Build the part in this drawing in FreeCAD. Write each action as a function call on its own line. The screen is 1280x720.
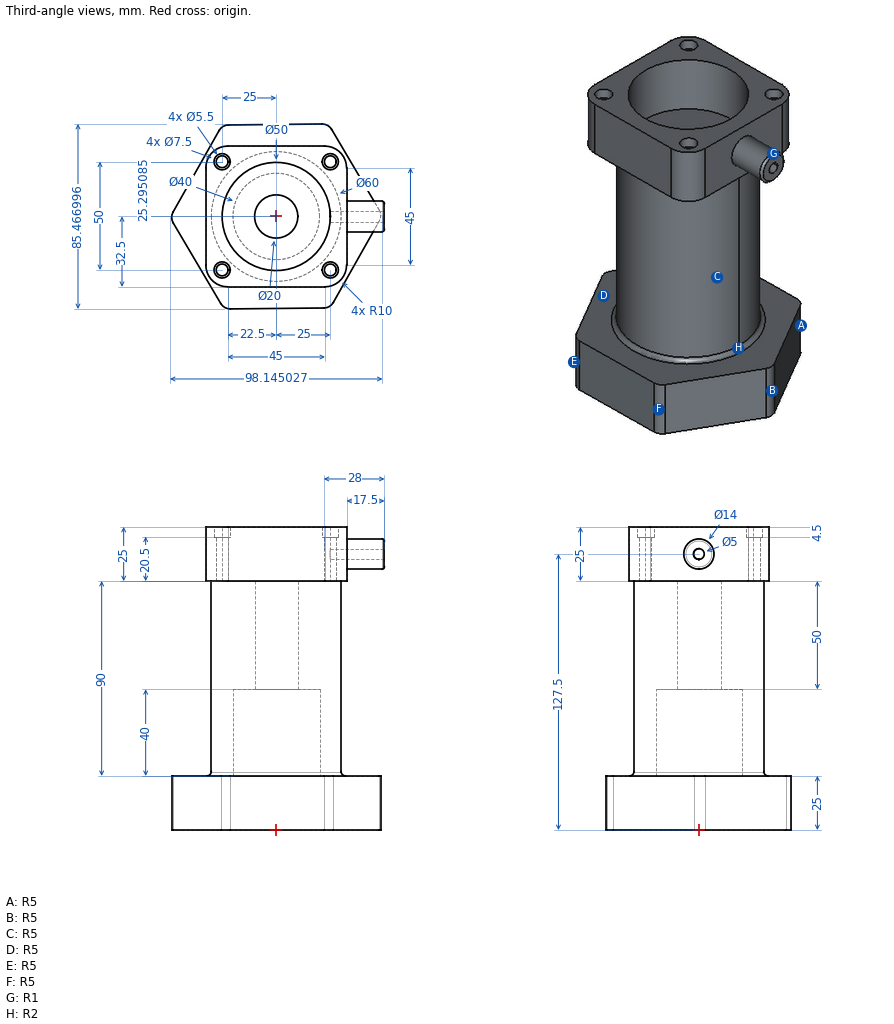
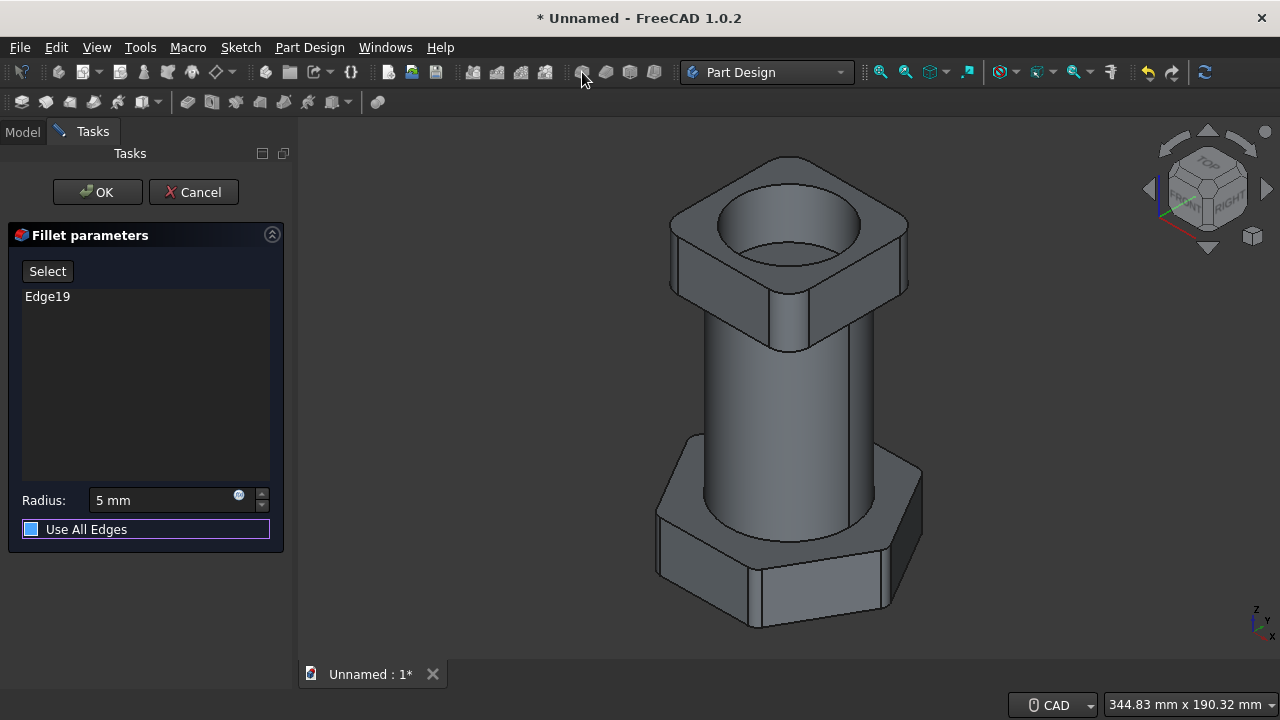
click(98, 192)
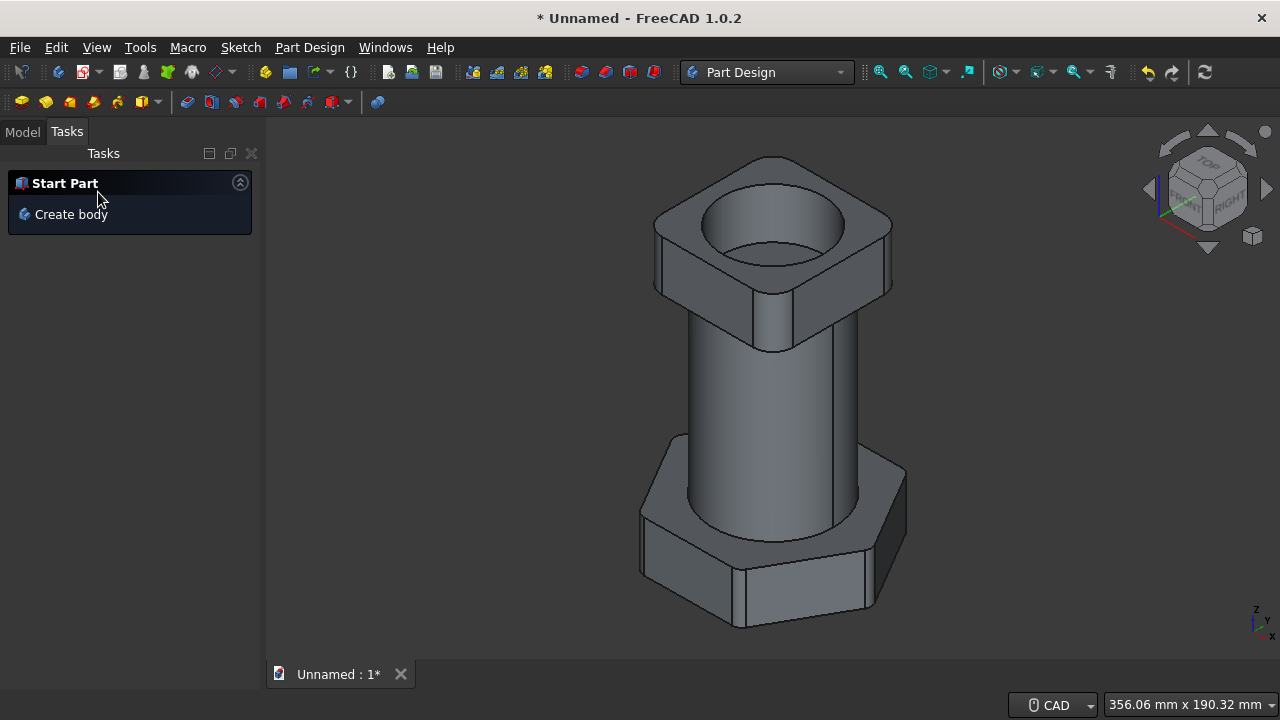
click(867, 235)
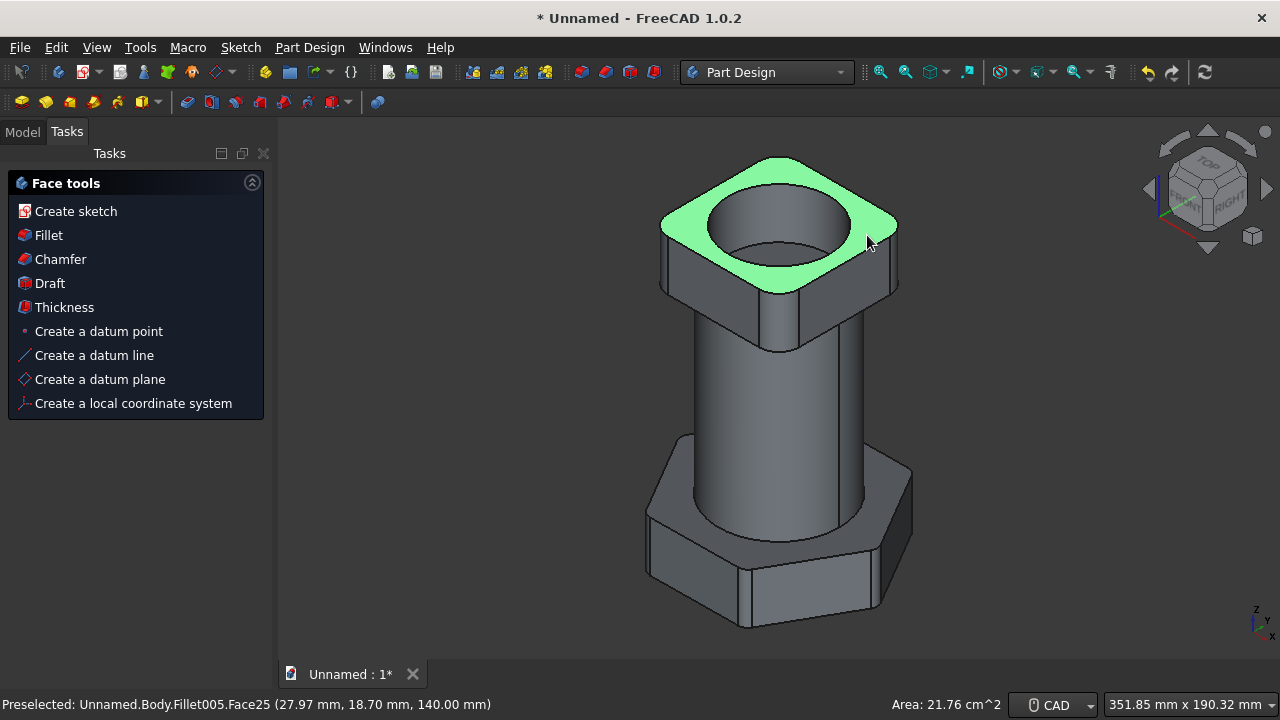
click(84, 72)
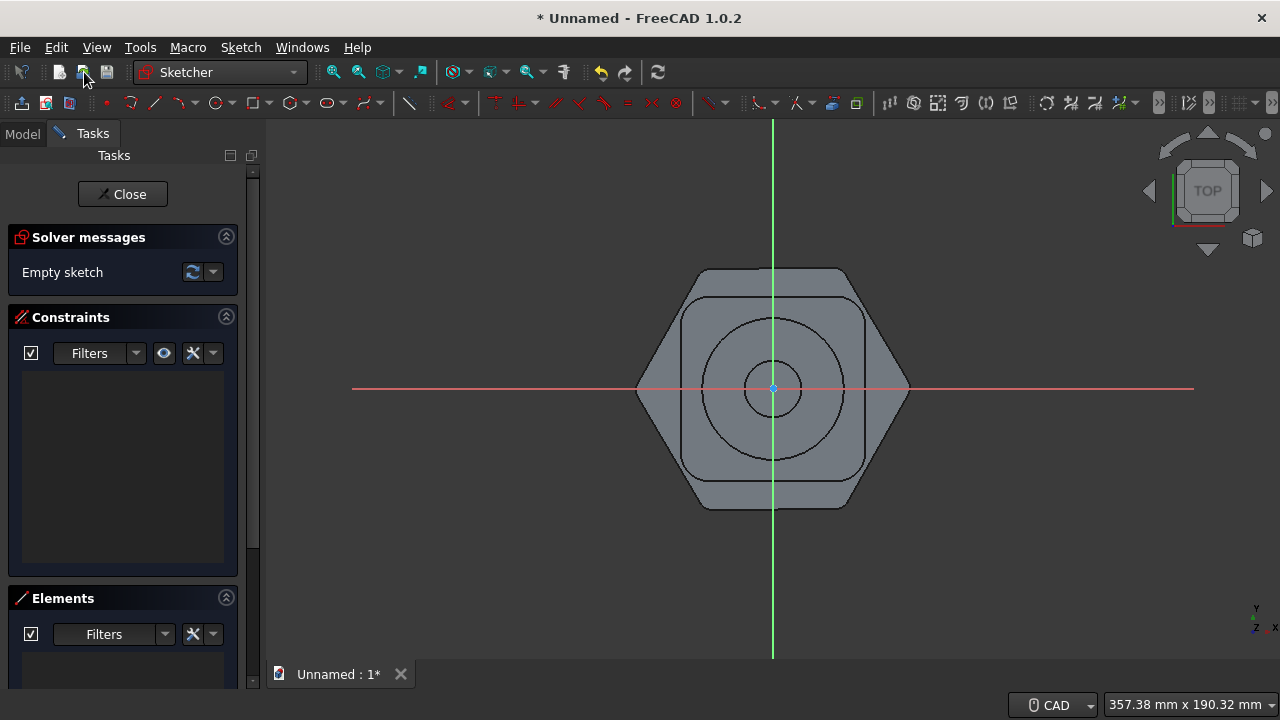
scroll(829, 387, up, 4)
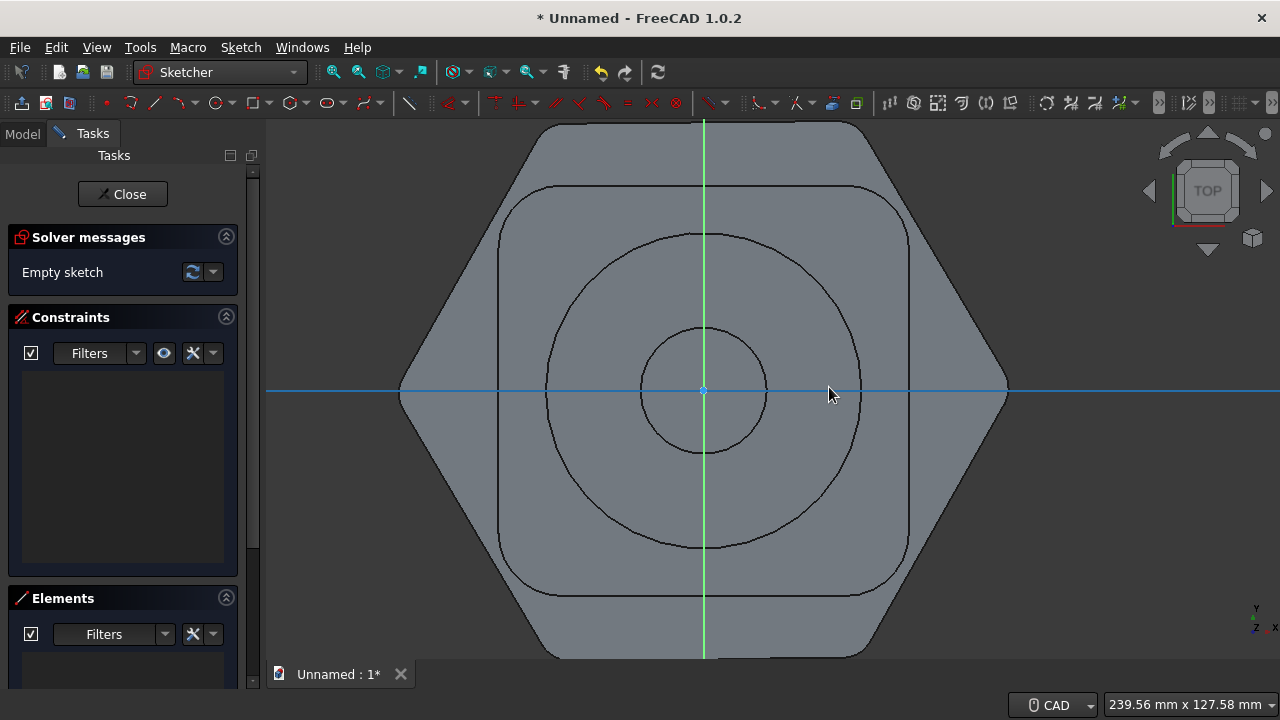
click(216, 104)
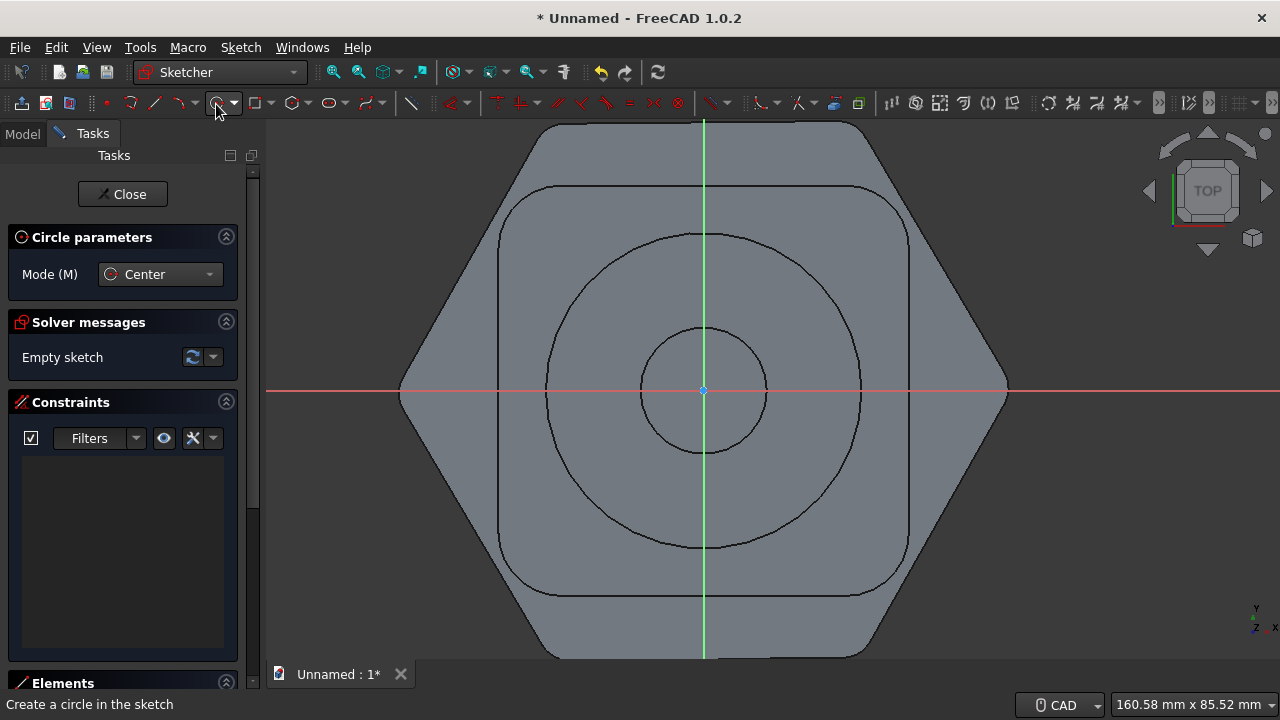
click(546, 231)
click(563, 214)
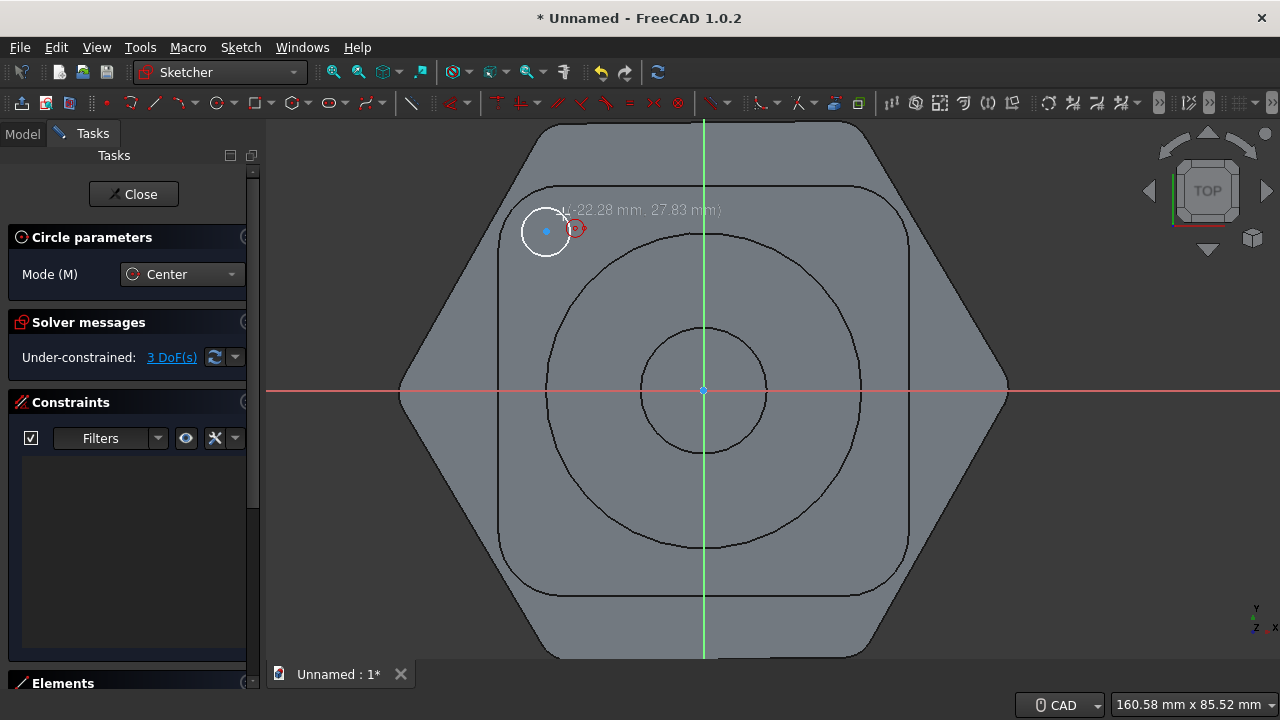
click(546, 547)
click(563, 530)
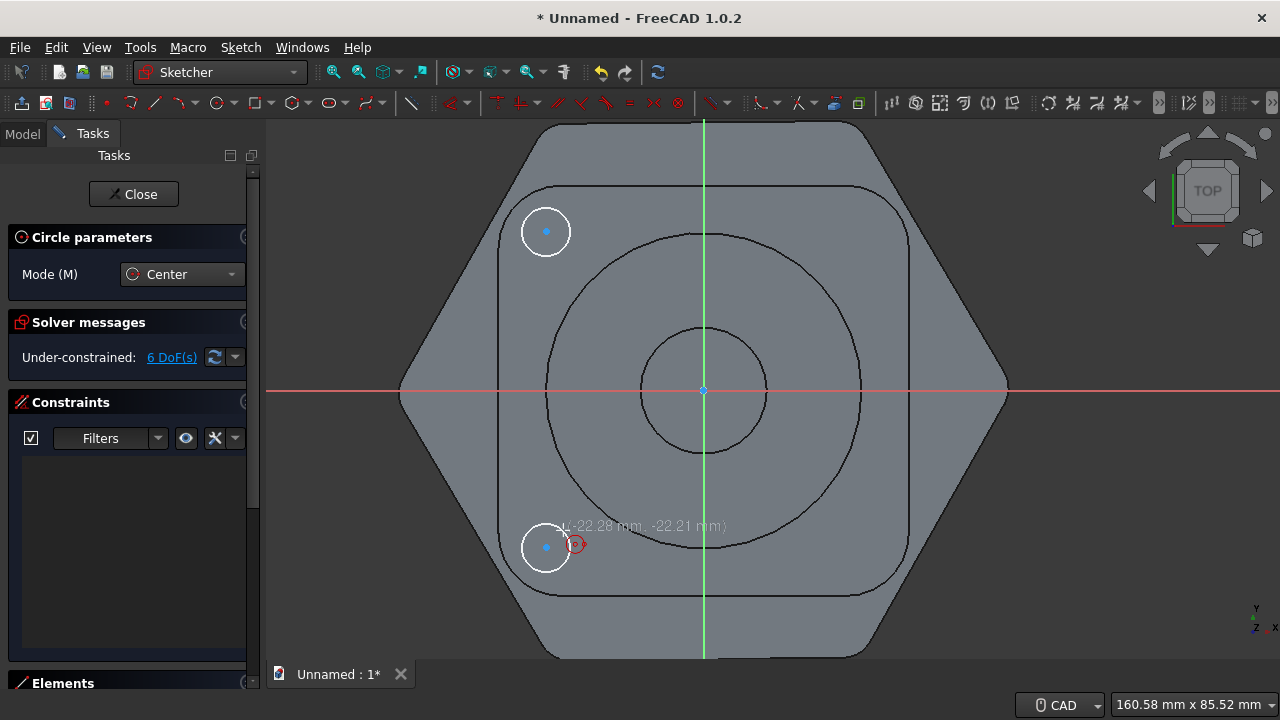
click(862, 547)
click(878, 530)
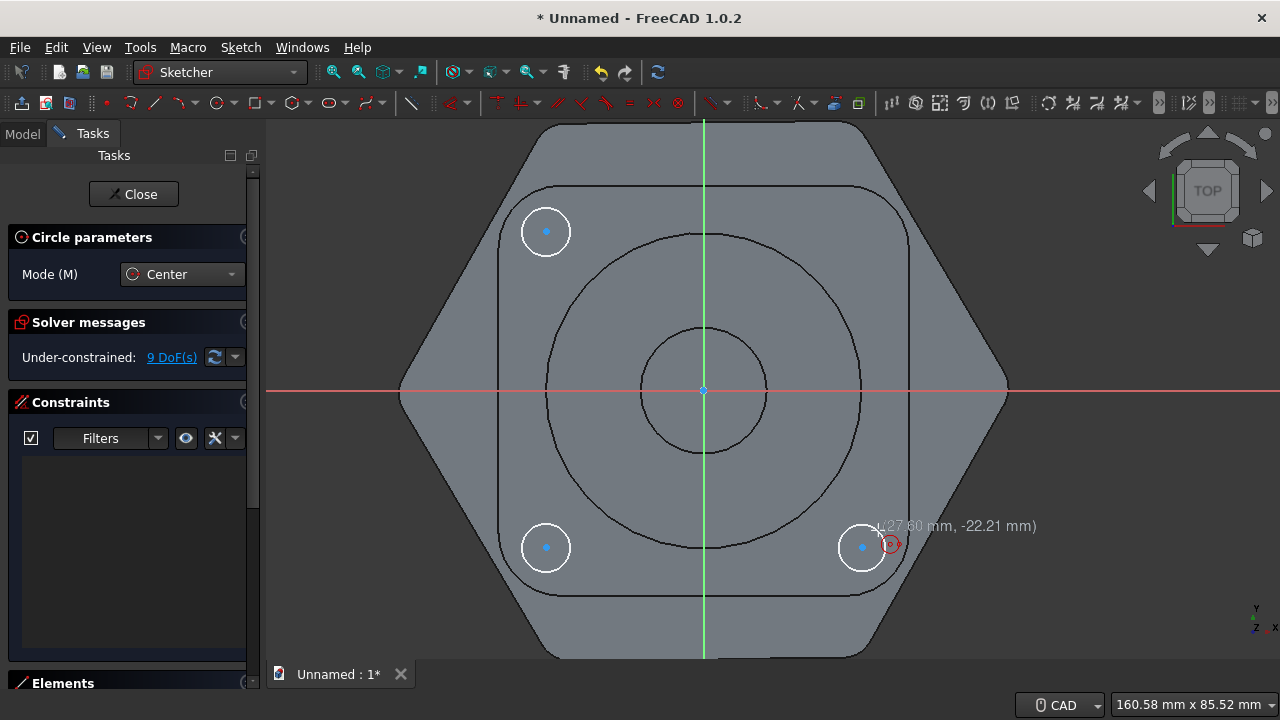
click(862, 231)
click(878, 214)
key(Escape)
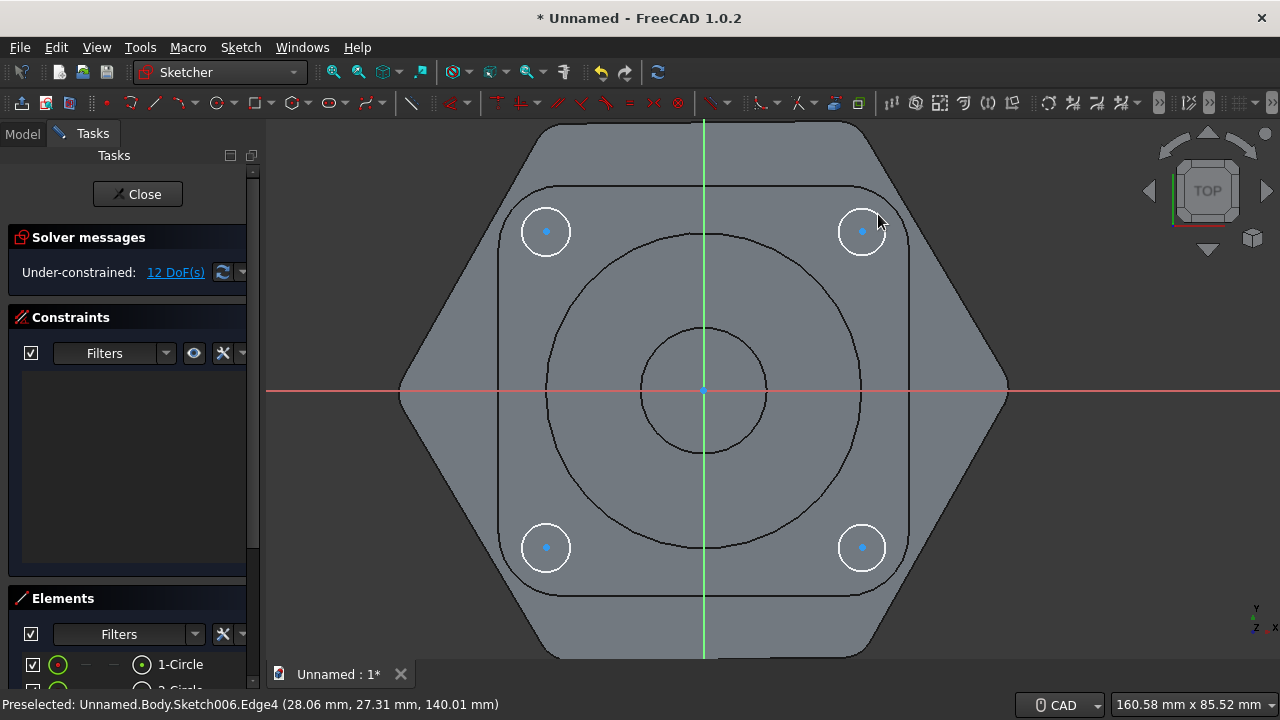
click(563, 215)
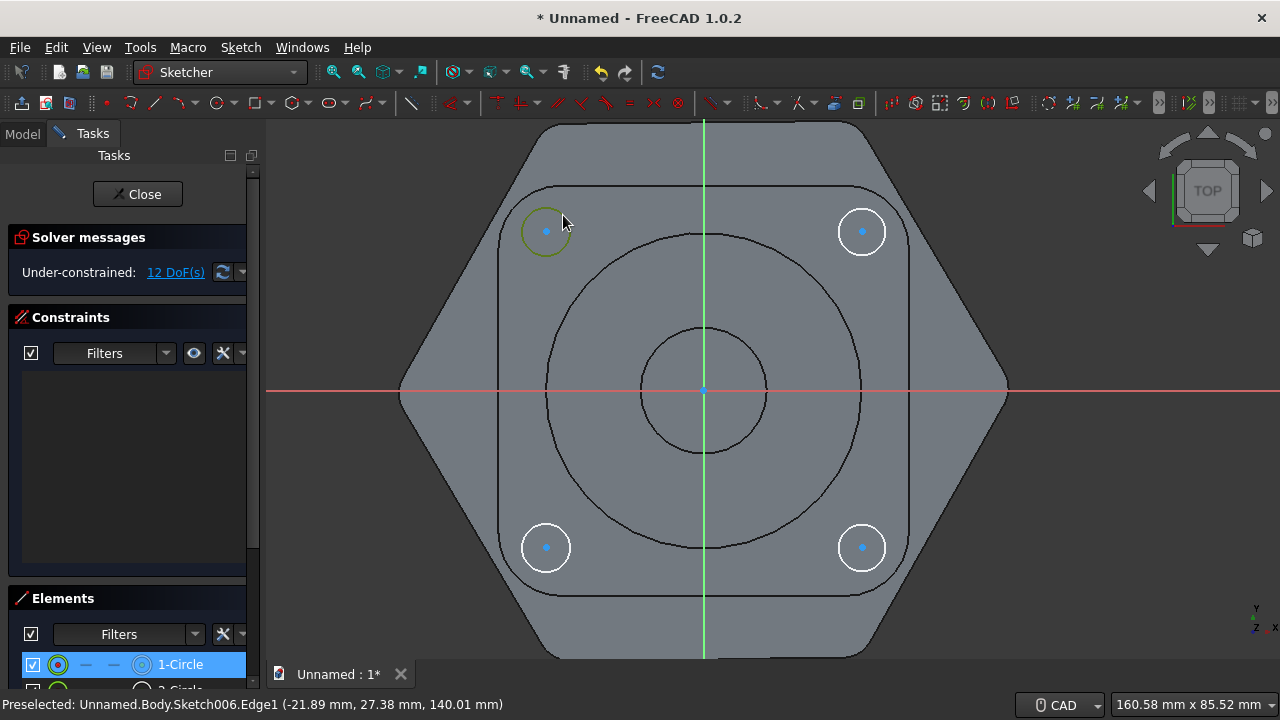
click(563, 531)